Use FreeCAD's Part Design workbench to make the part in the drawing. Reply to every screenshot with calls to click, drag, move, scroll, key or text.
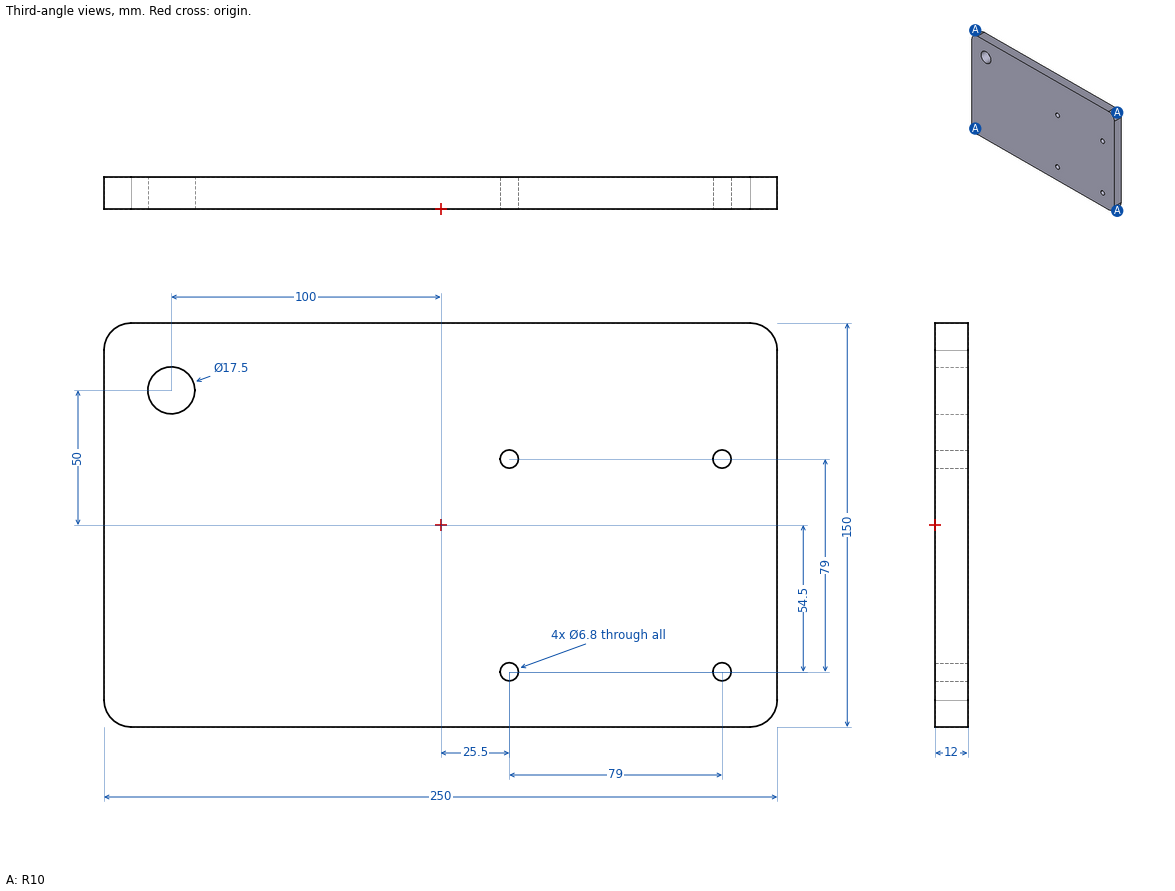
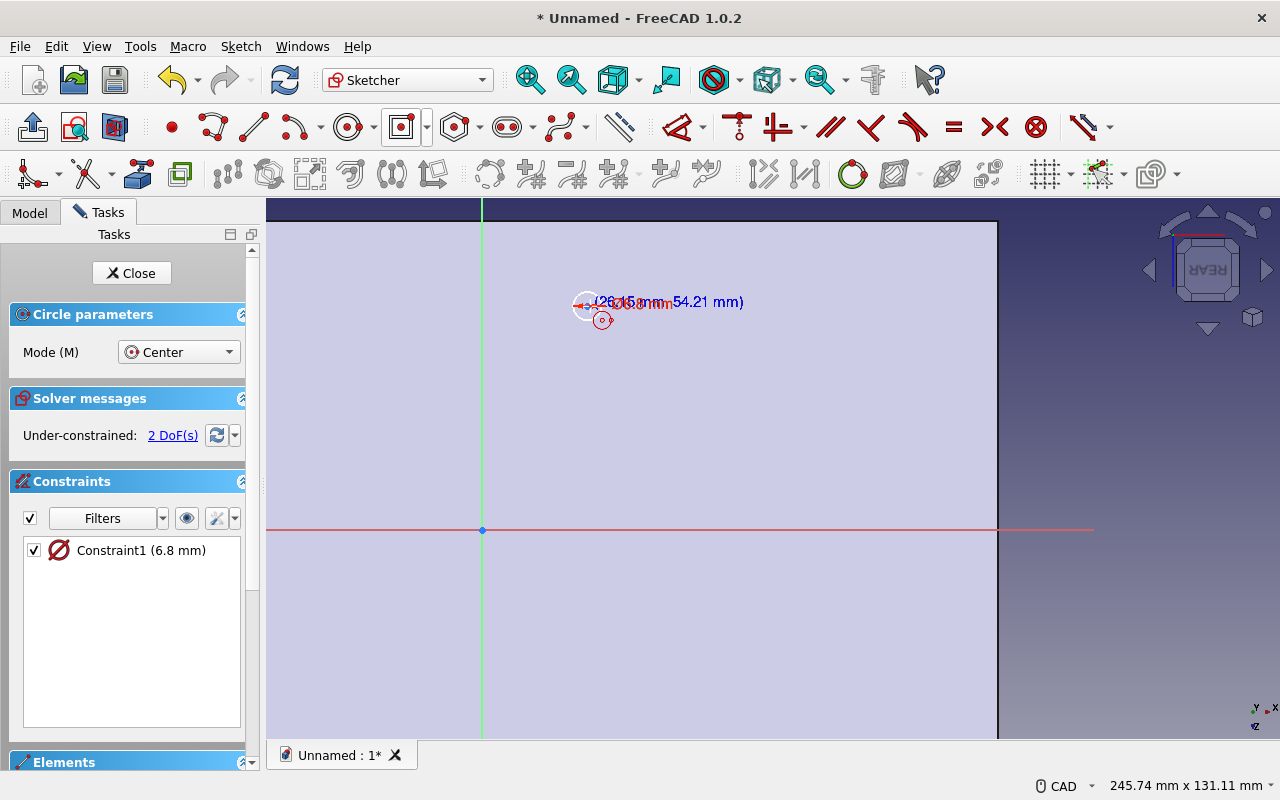
scroll(913, 305, up, 3)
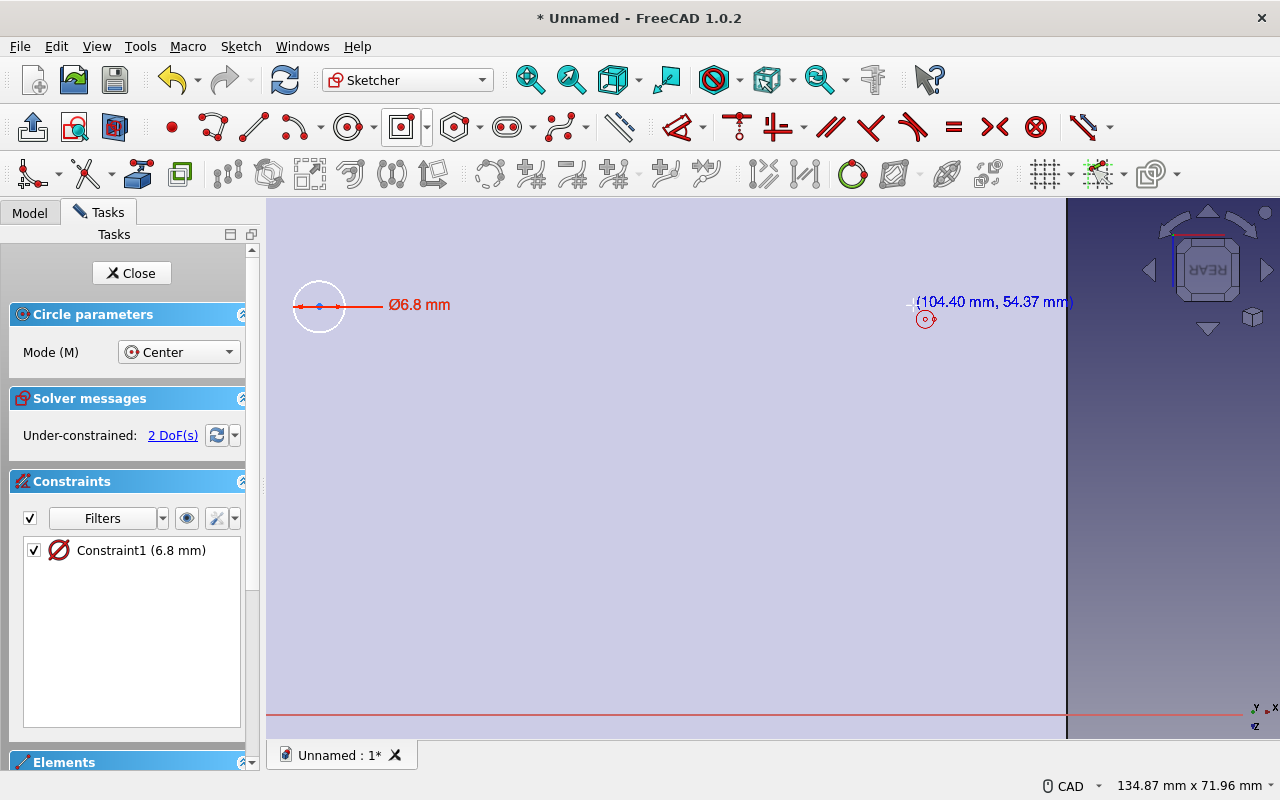
click(913, 306)
move(931, 288)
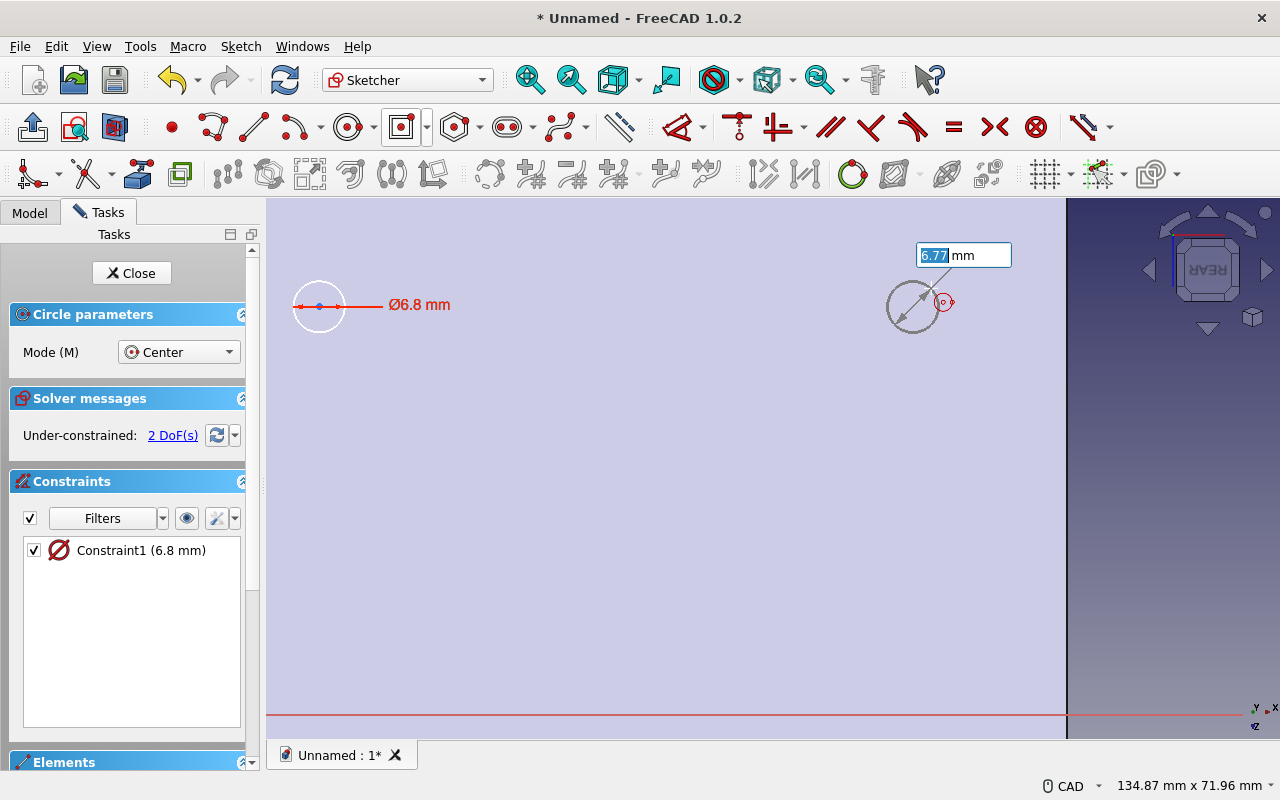
text(6.8)
key(Return)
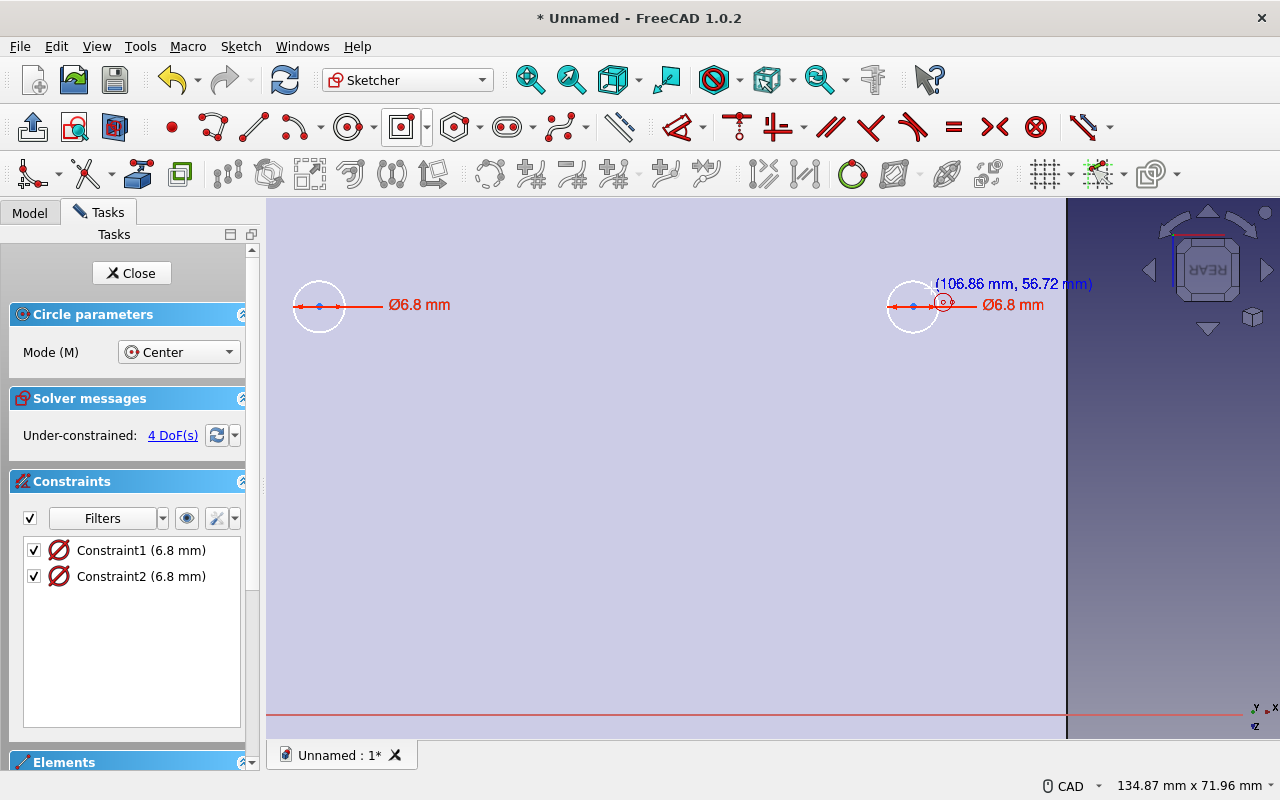
scroll(913, 305, down, 3)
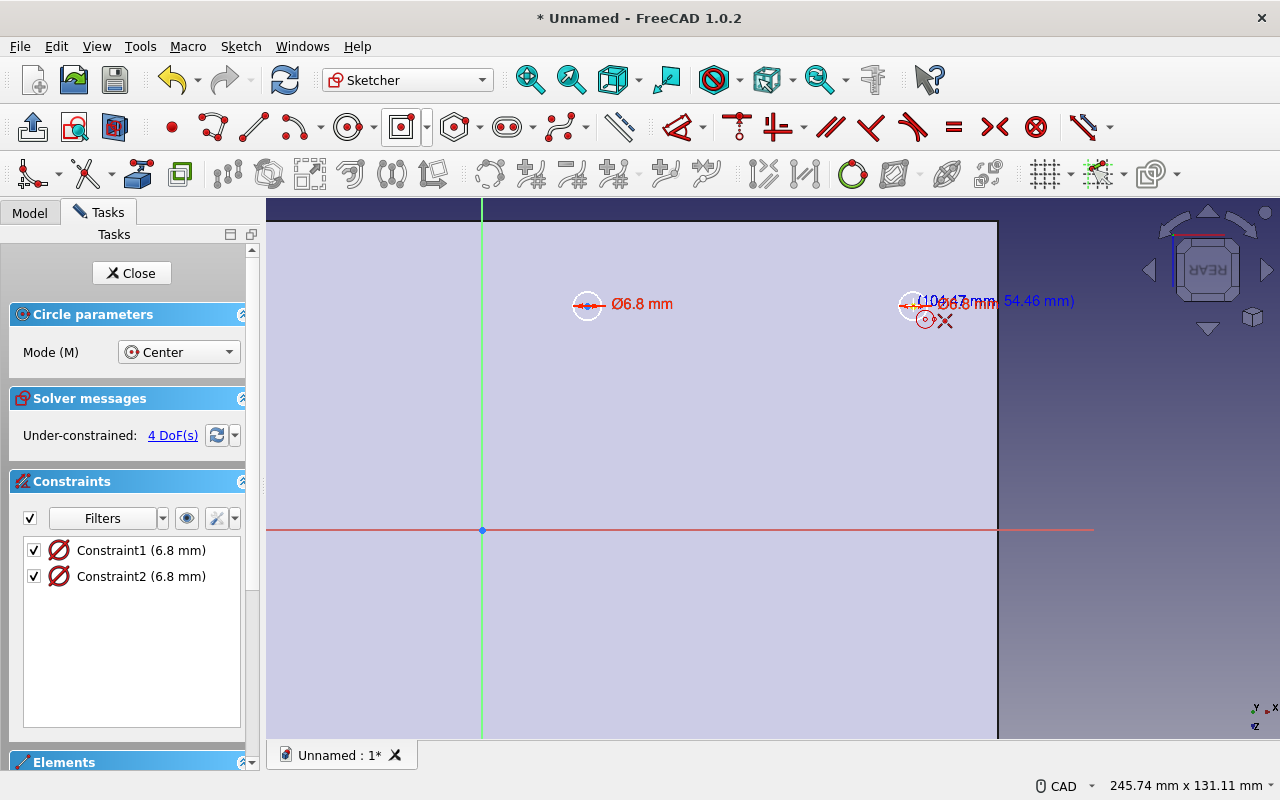
scroll(587, 631, up, 3)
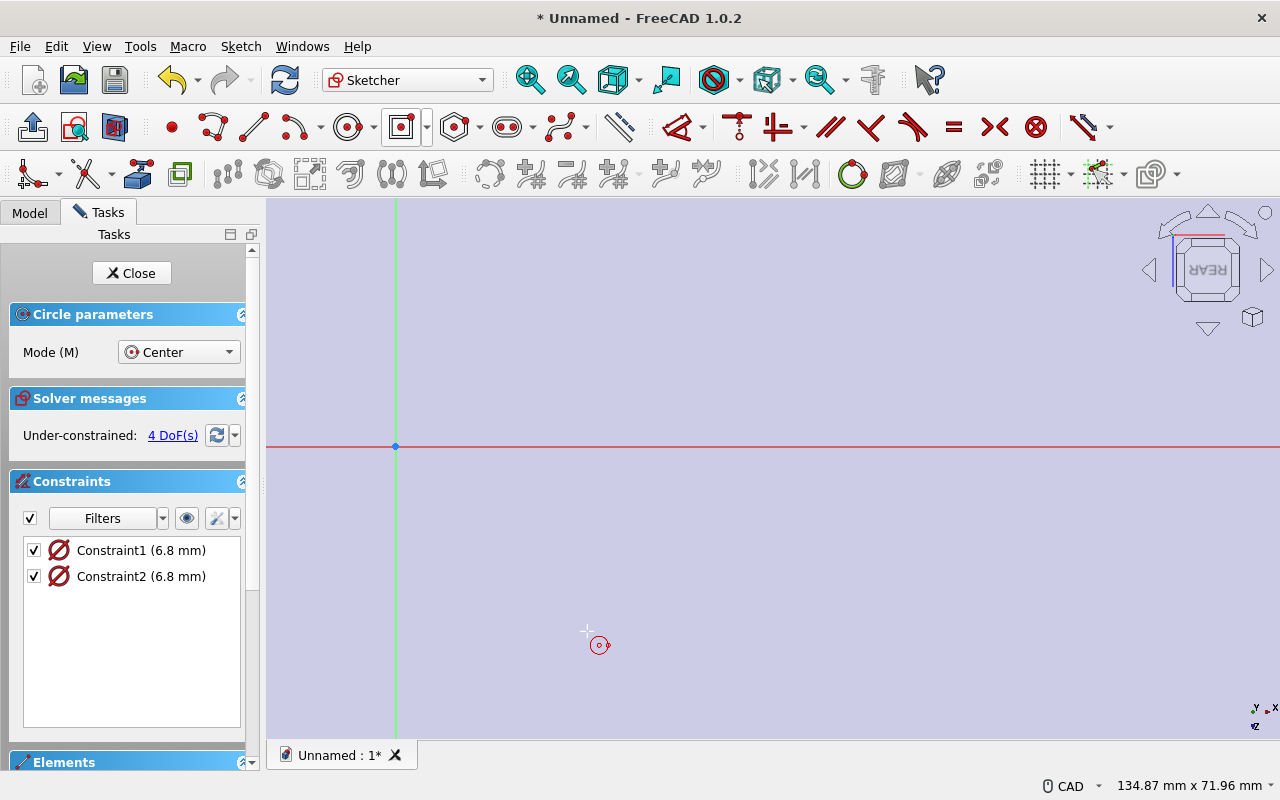
click(588, 631)
move(606, 613)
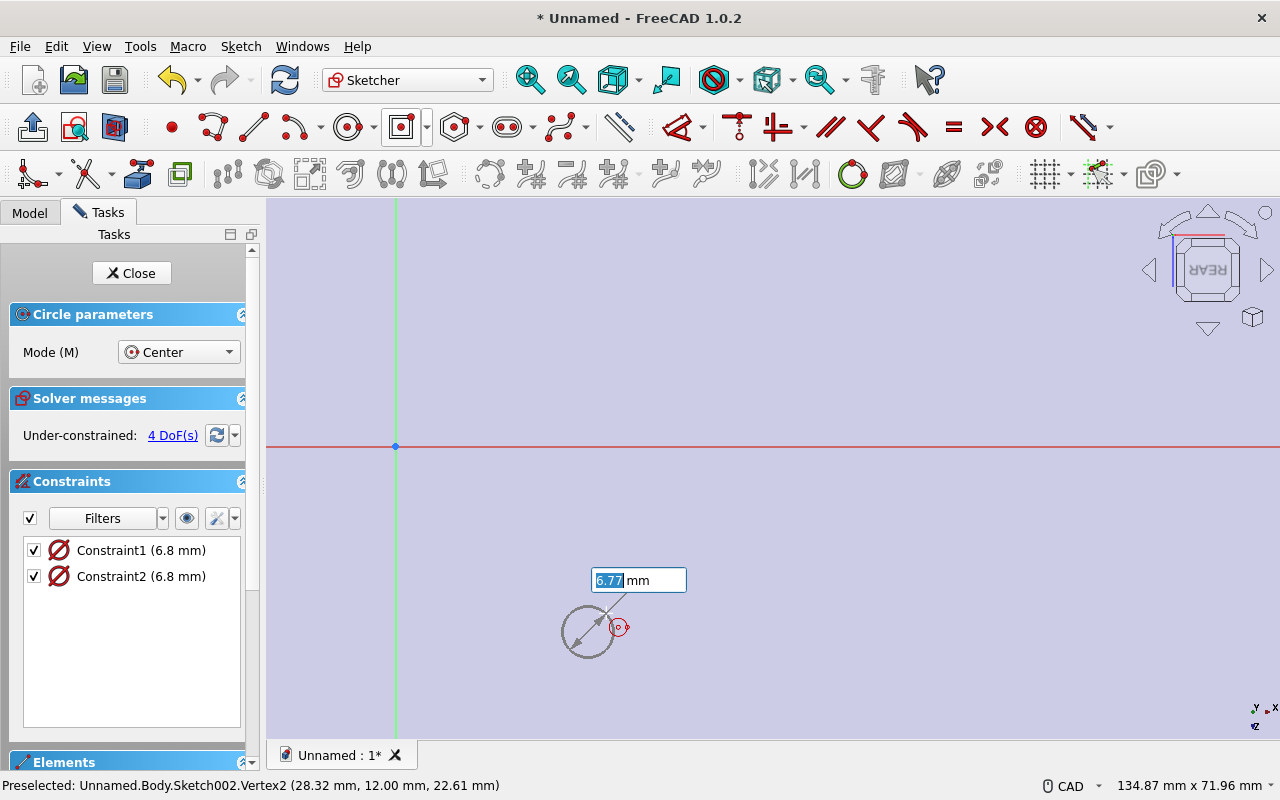
text(6.8)
key(Return)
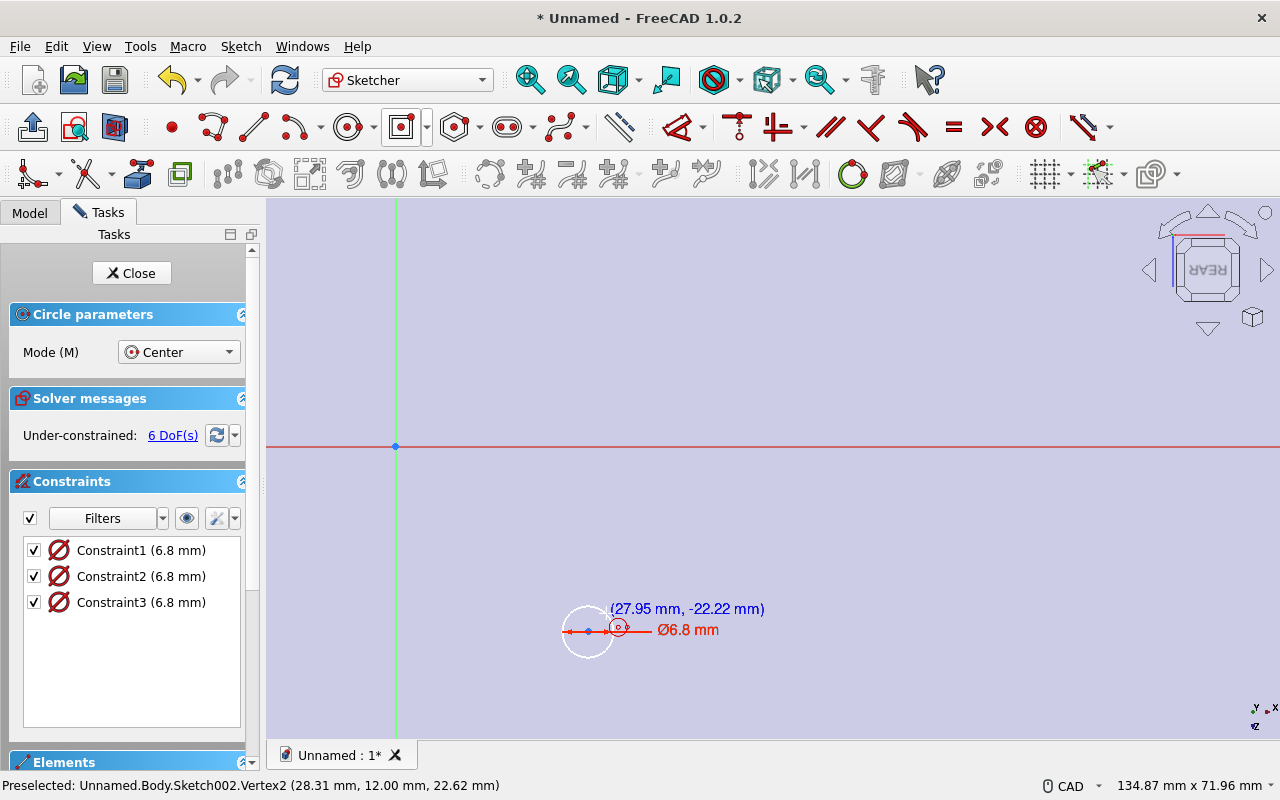
scroll(587, 632, down, 3)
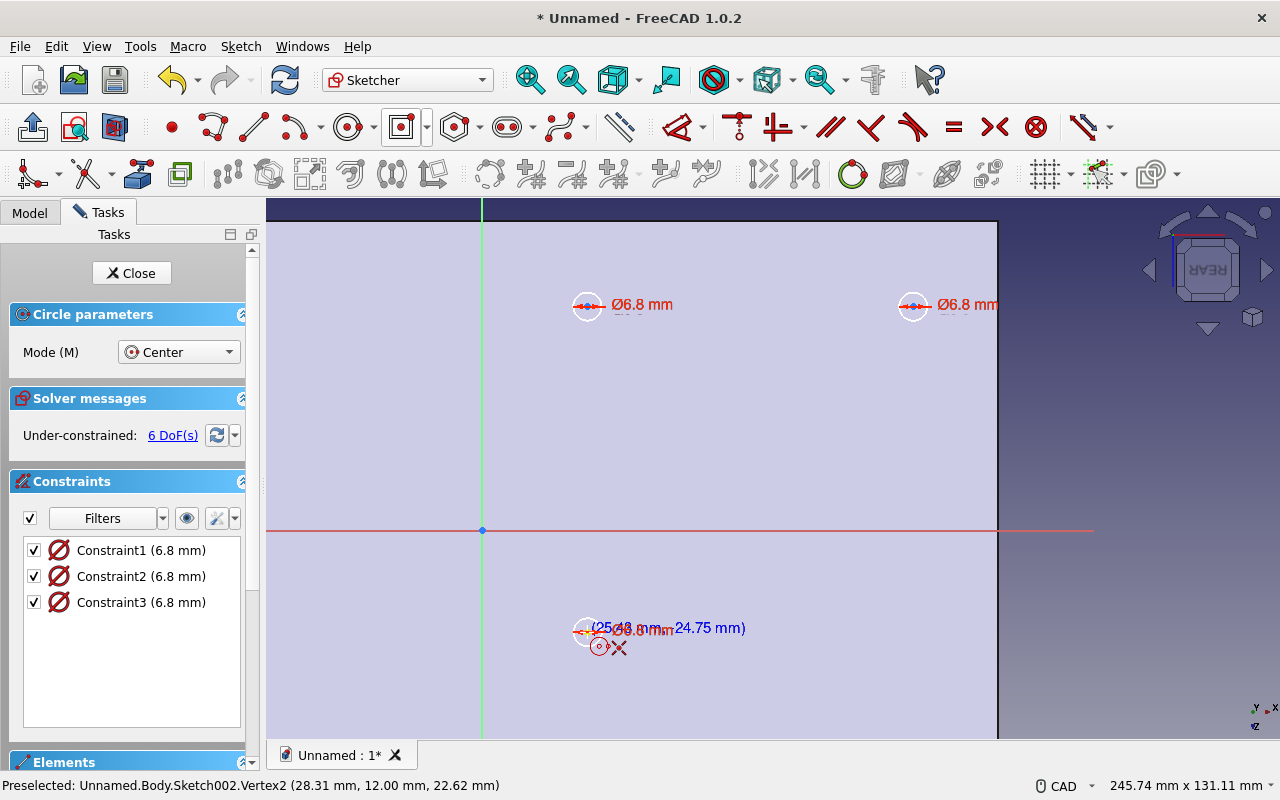
scroll(913, 632, up, 3)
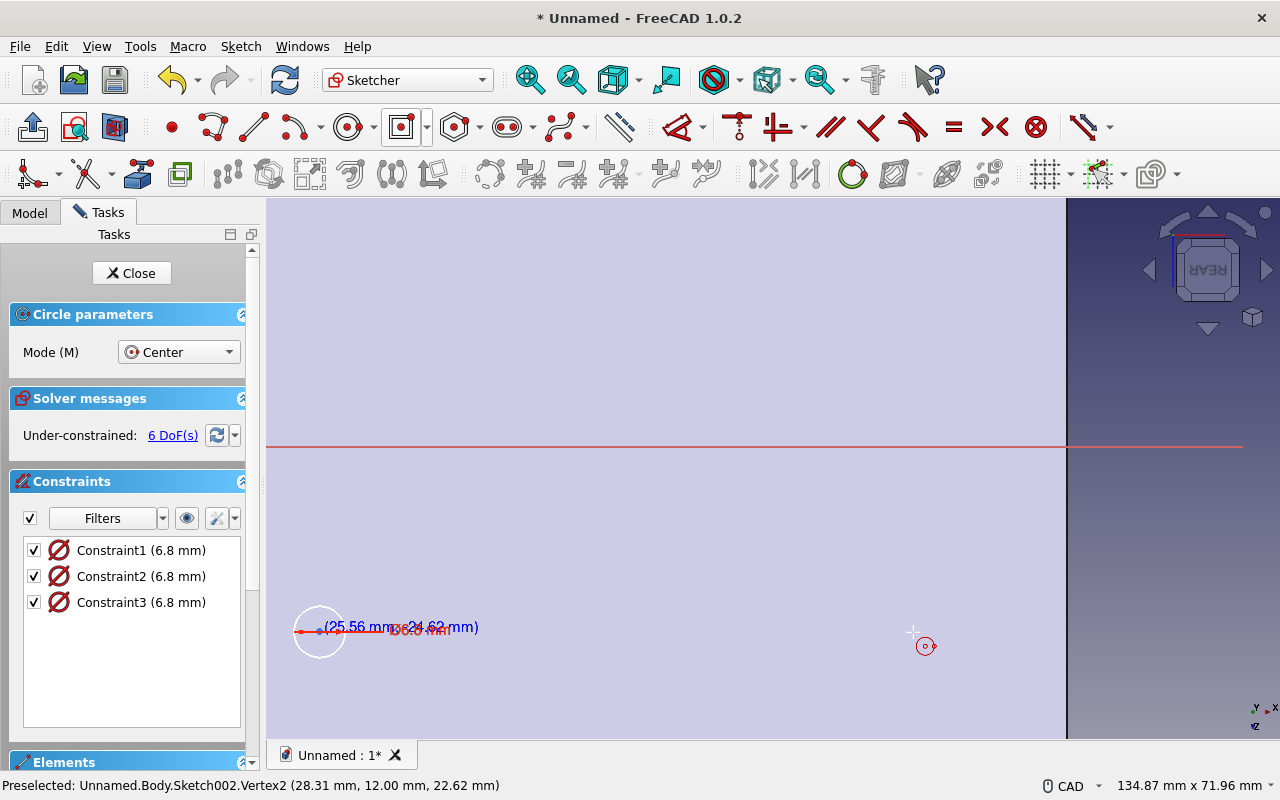
click(913, 631)
move(931, 613)